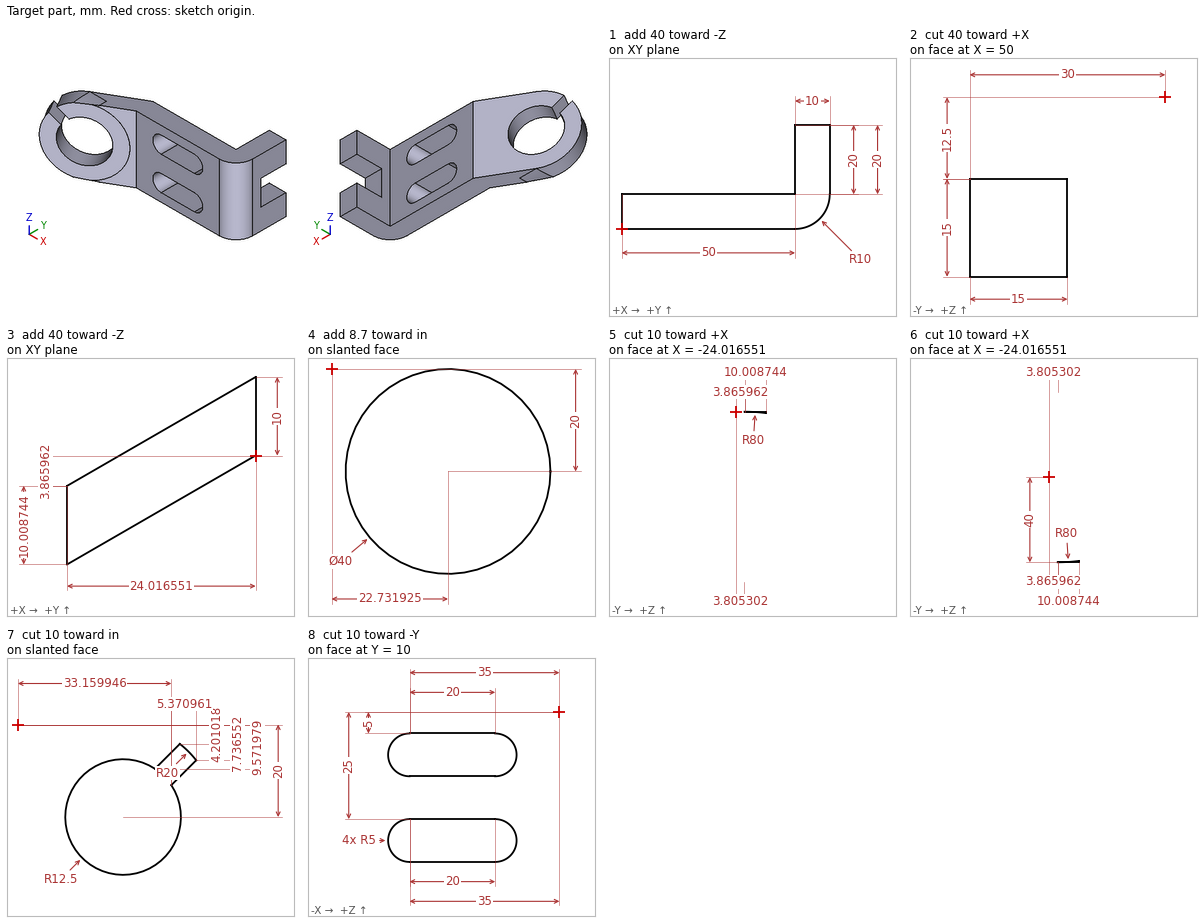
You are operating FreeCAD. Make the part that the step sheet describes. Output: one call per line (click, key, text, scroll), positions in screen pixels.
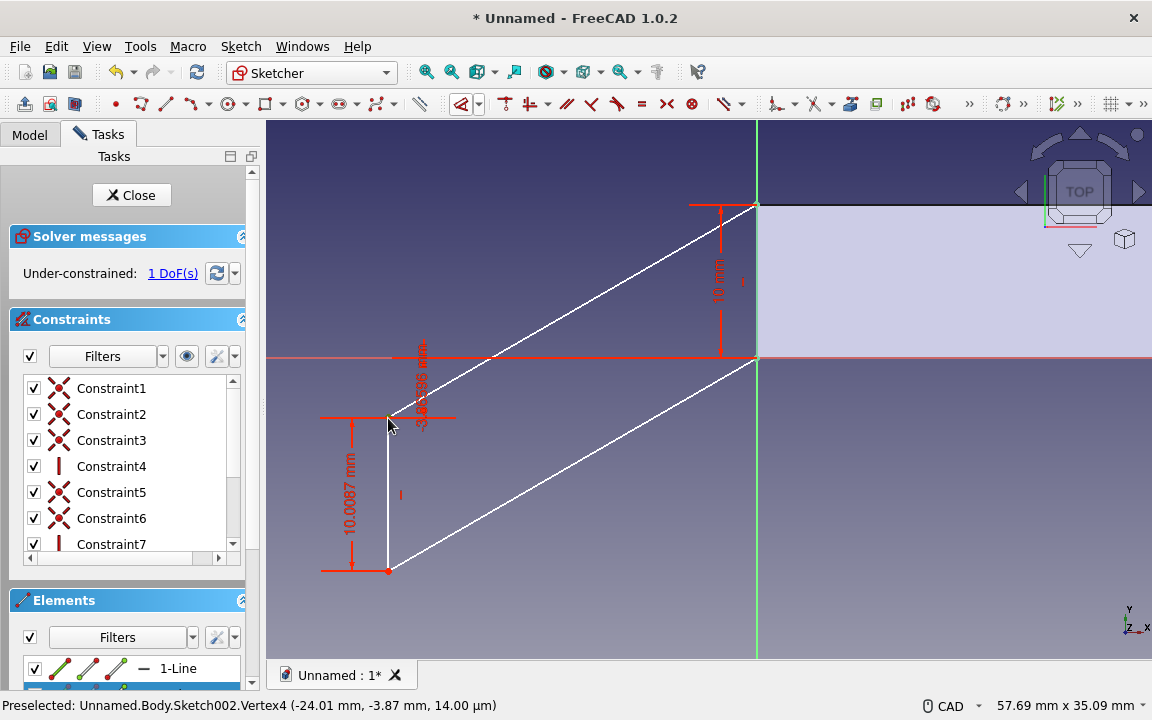
key(l)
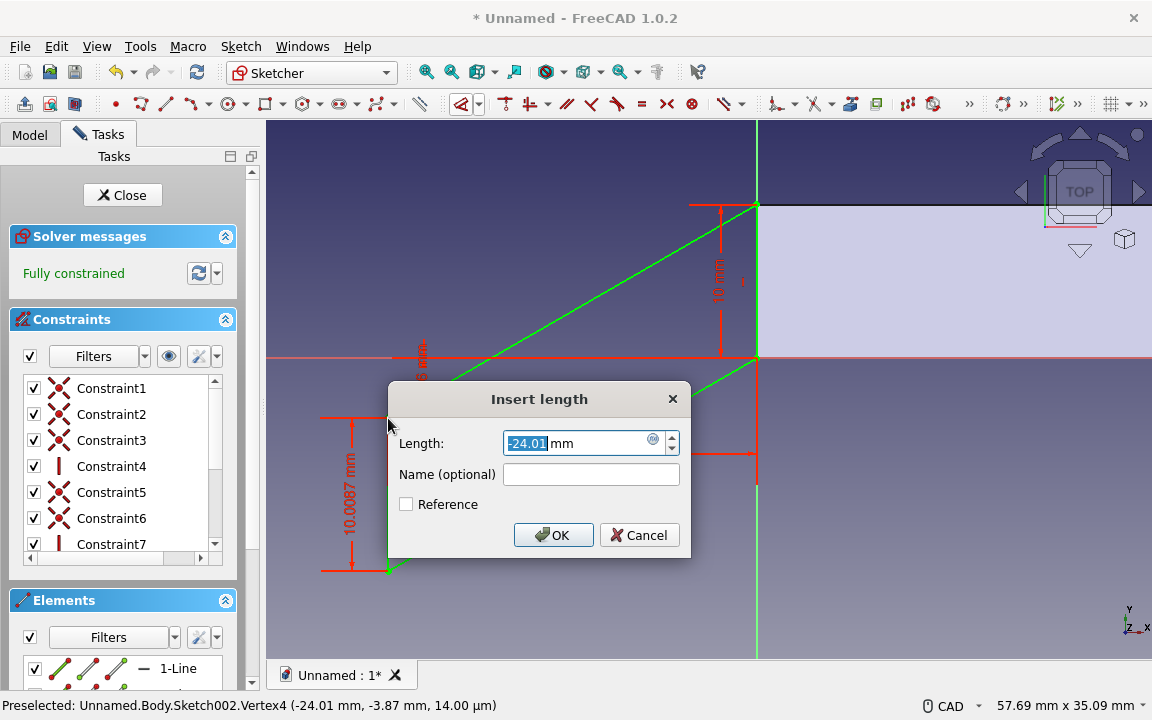
text(-24.016551)
key(Return)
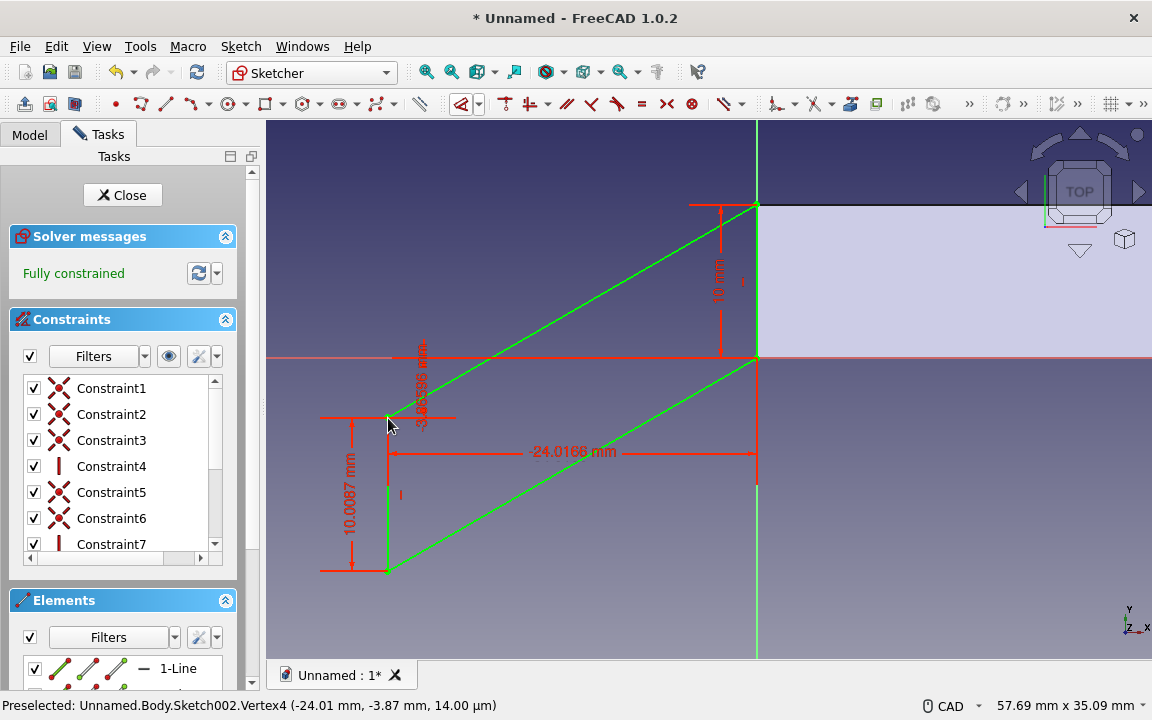
click(123, 195)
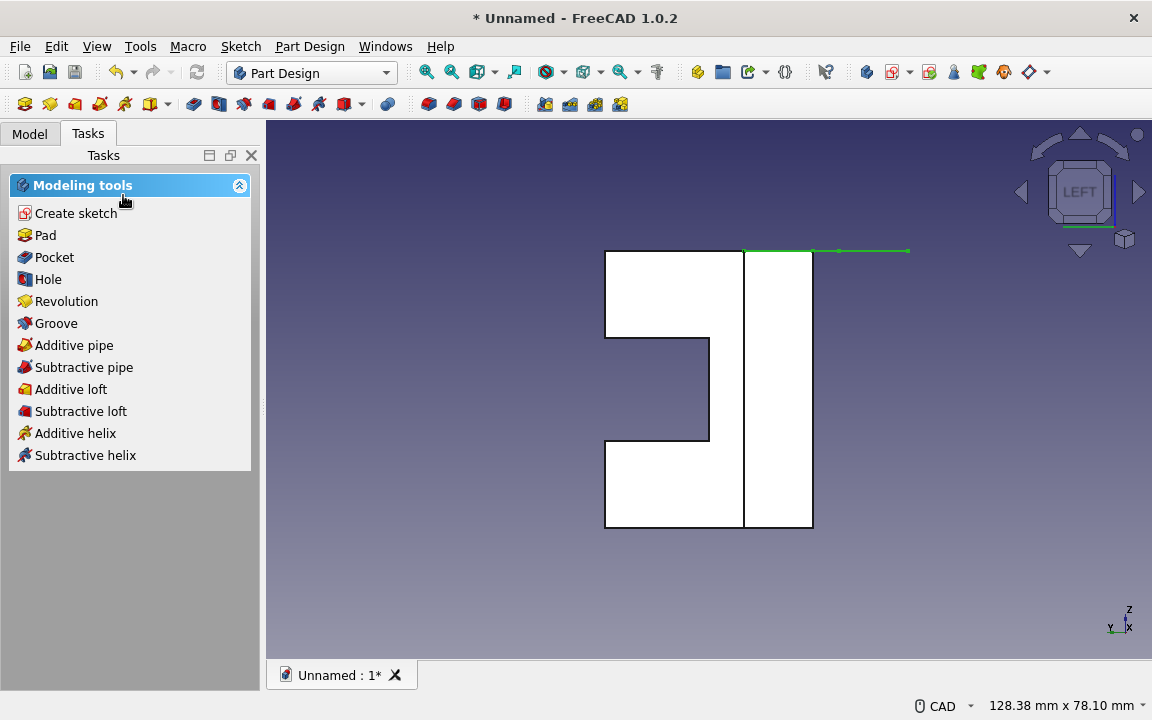
click(25, 104)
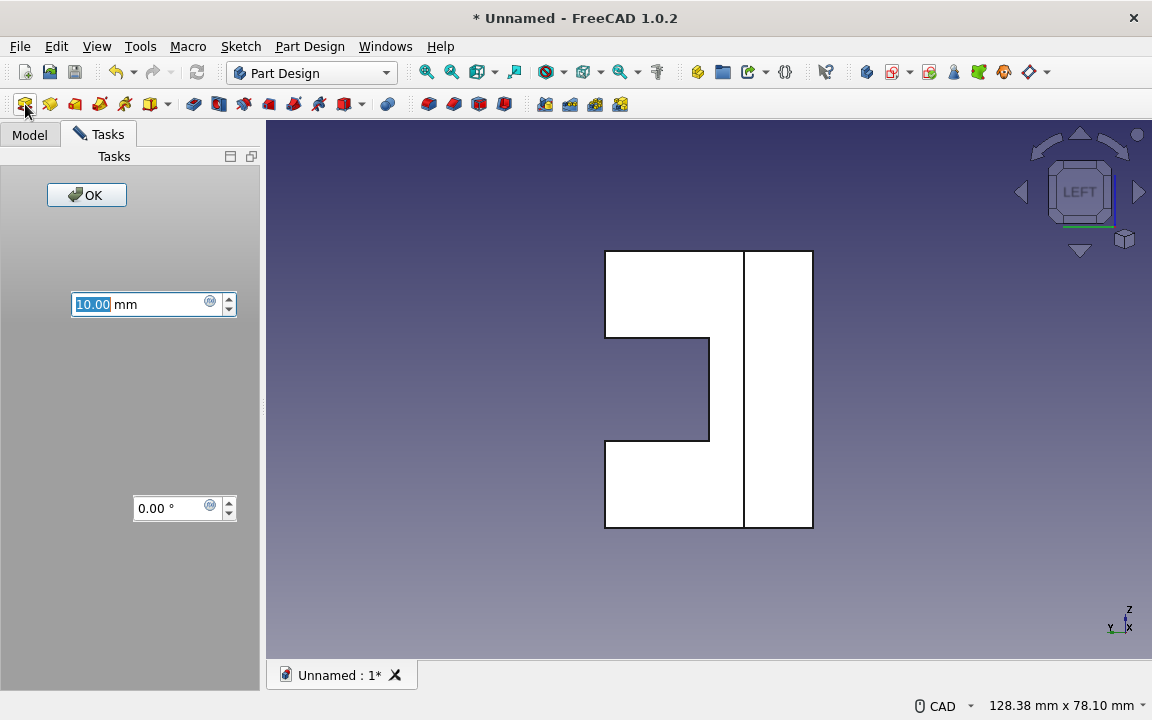
text(40)
key(Tab)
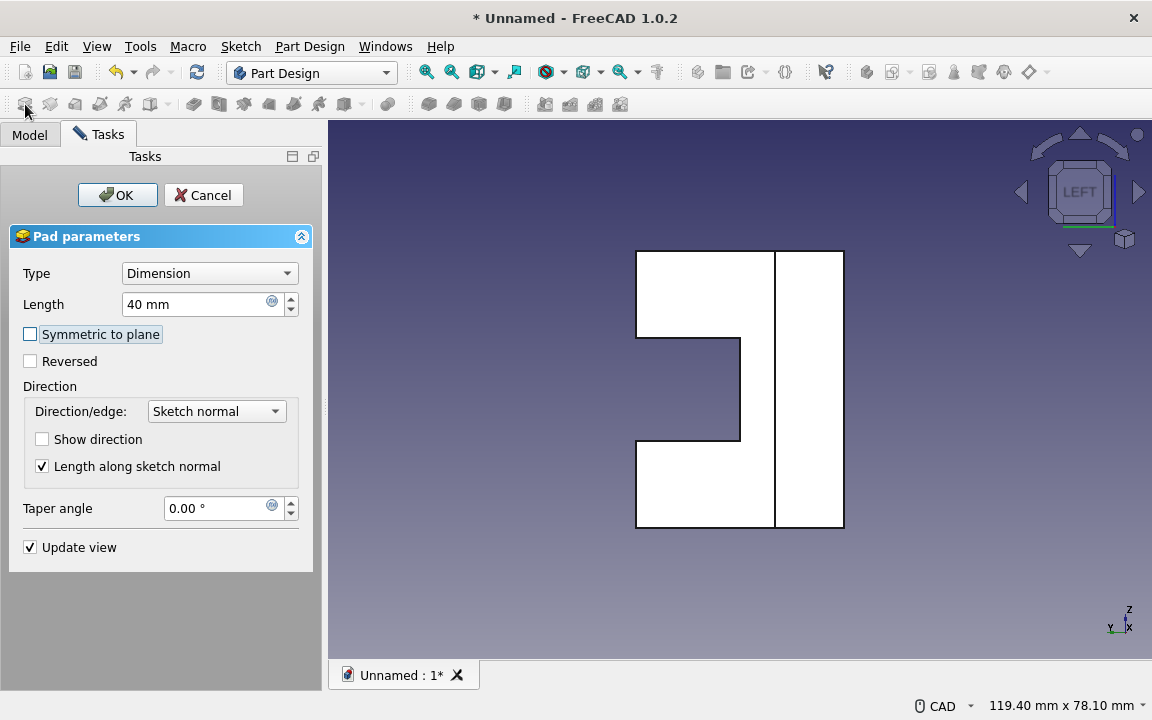
click(31, 361)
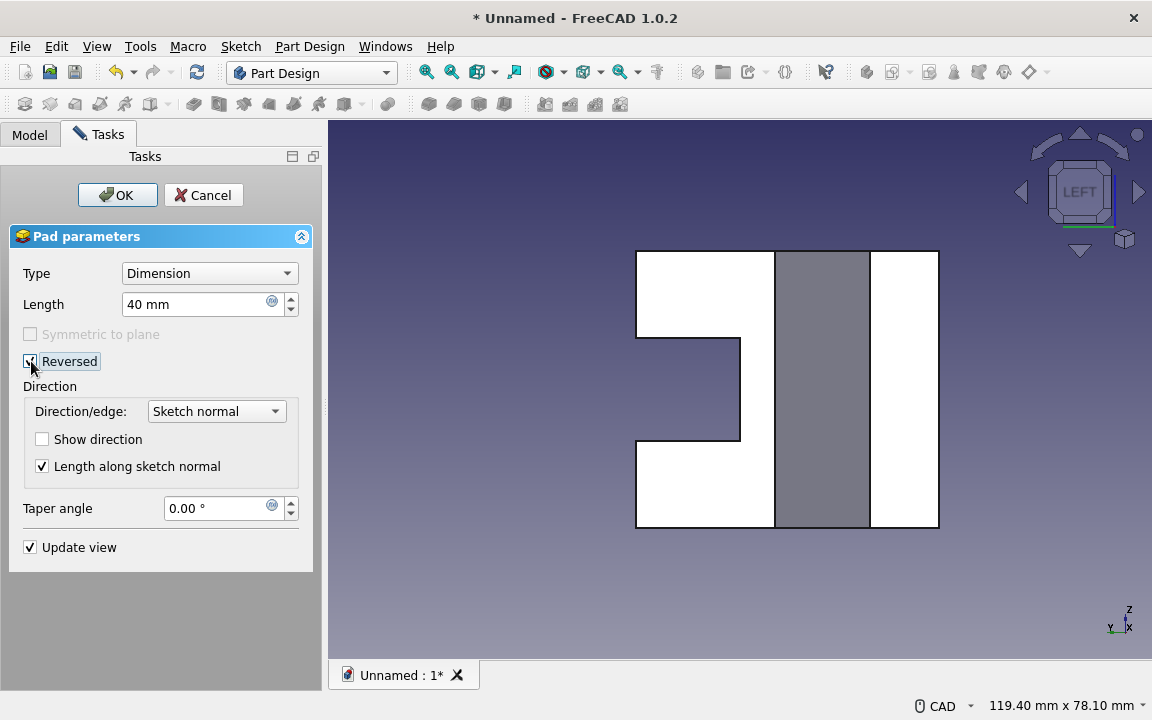
click(118, 195)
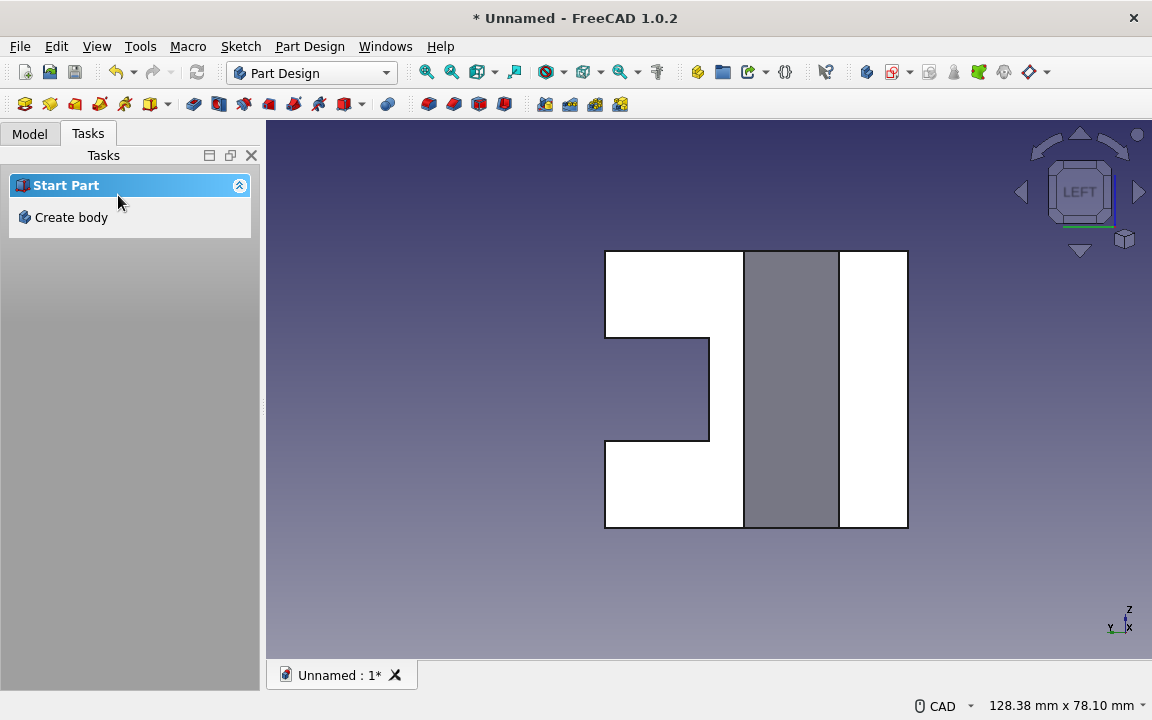
click(791, 349)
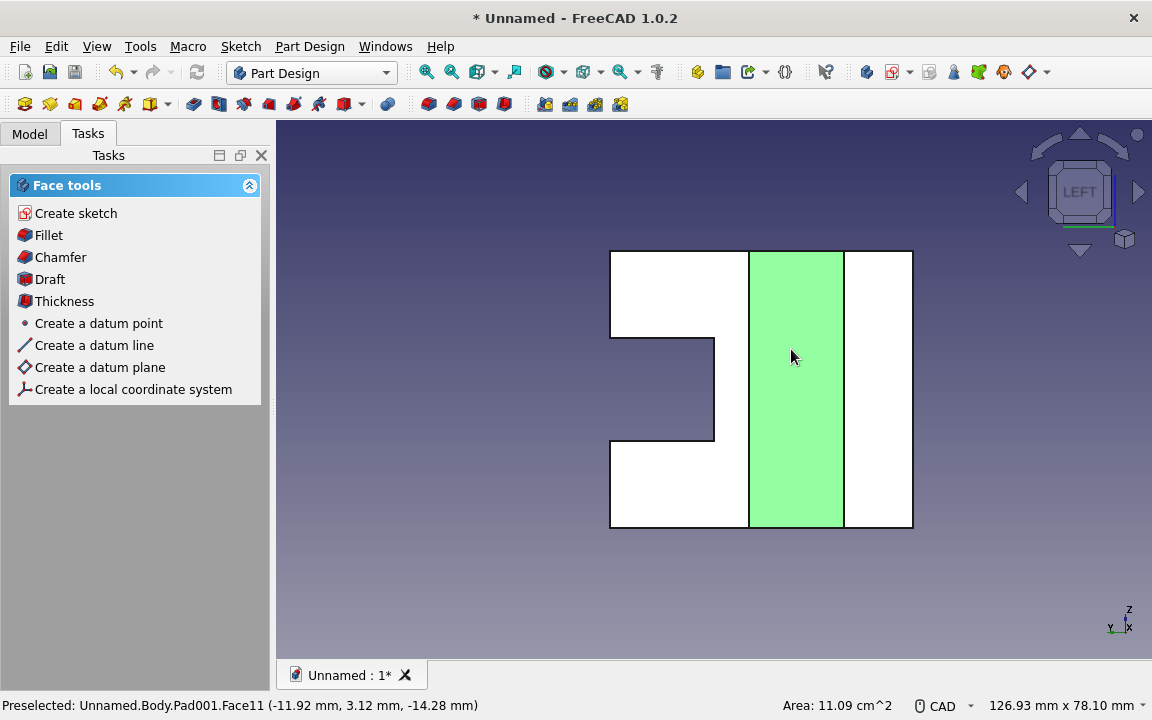
click(892, 72)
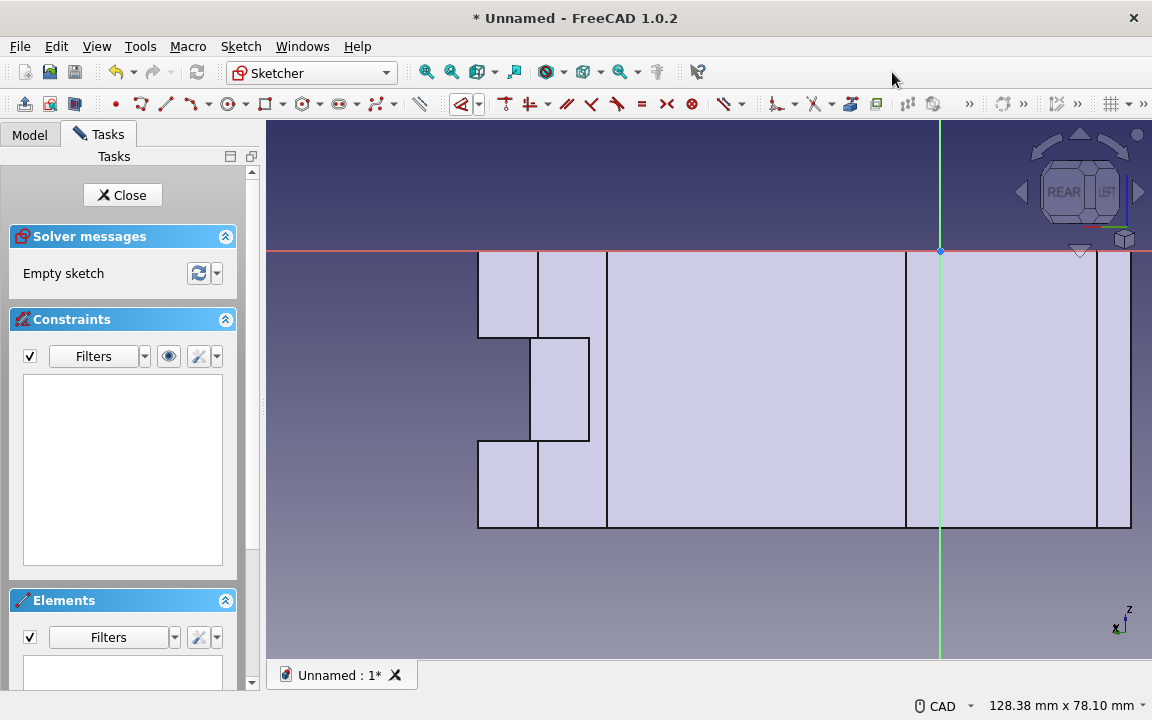
scroll(294, 389, down, 2)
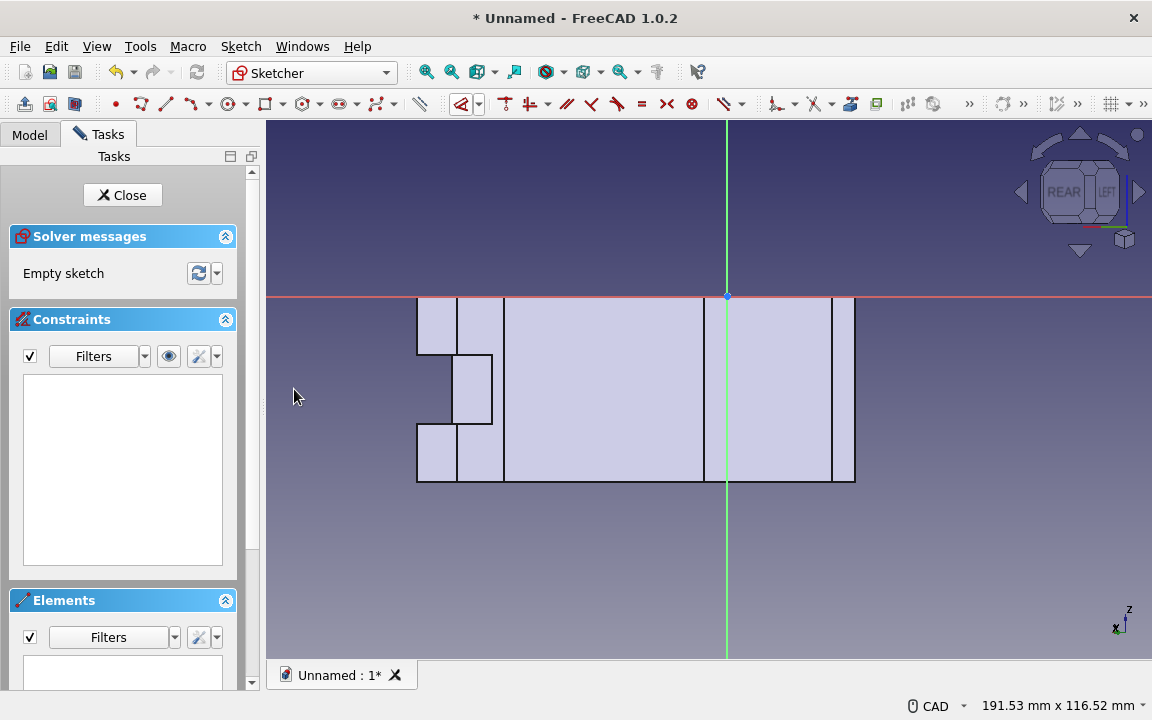
scroll(987, 390, up, 3)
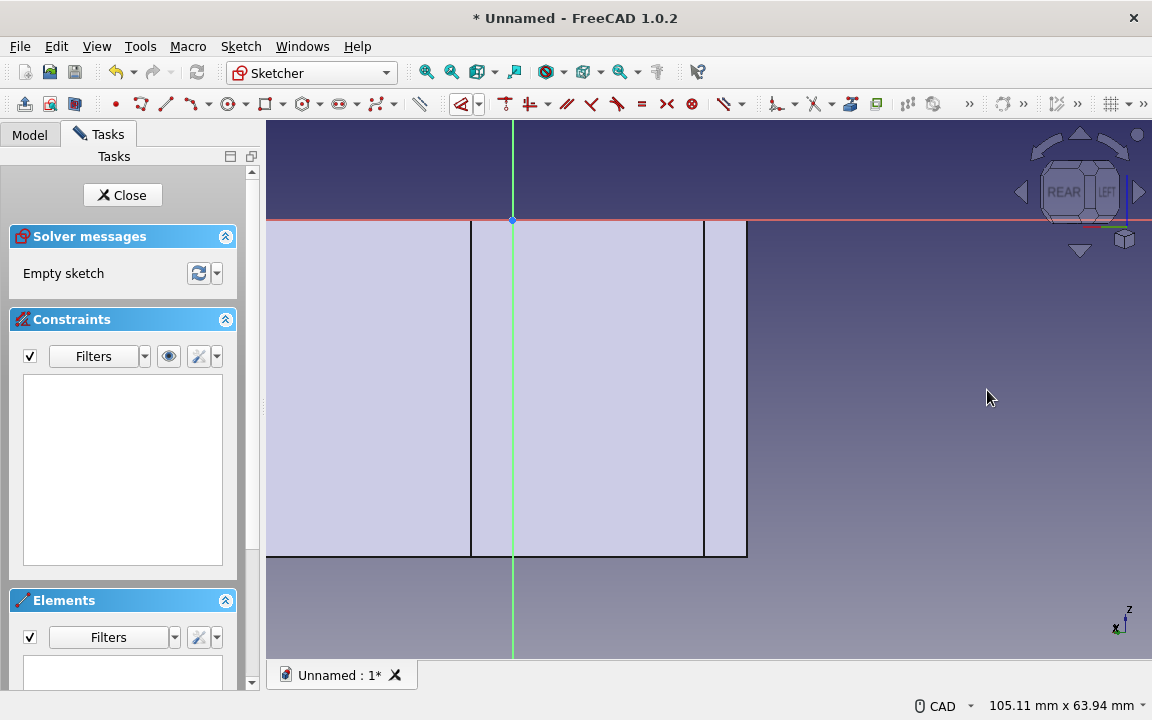
click(228, 104)